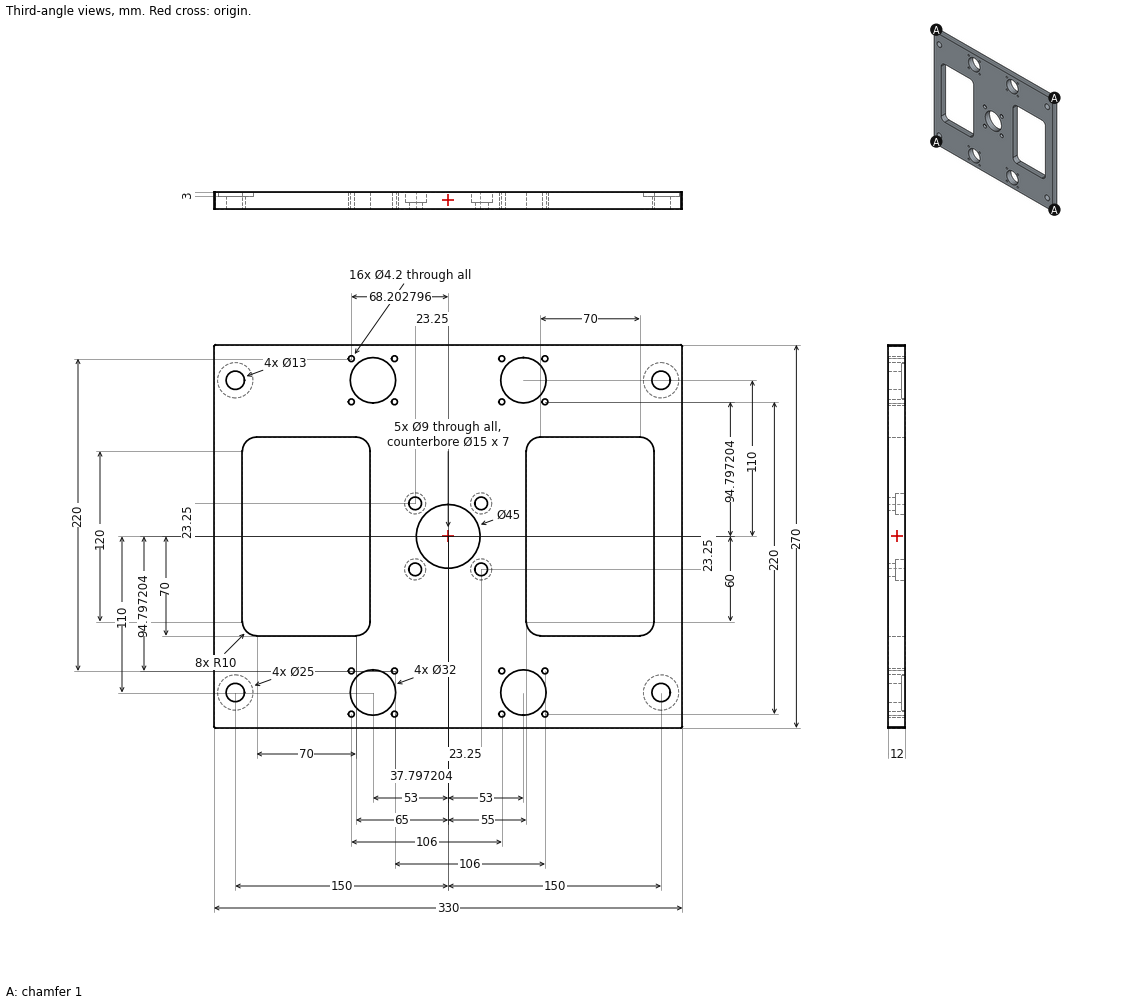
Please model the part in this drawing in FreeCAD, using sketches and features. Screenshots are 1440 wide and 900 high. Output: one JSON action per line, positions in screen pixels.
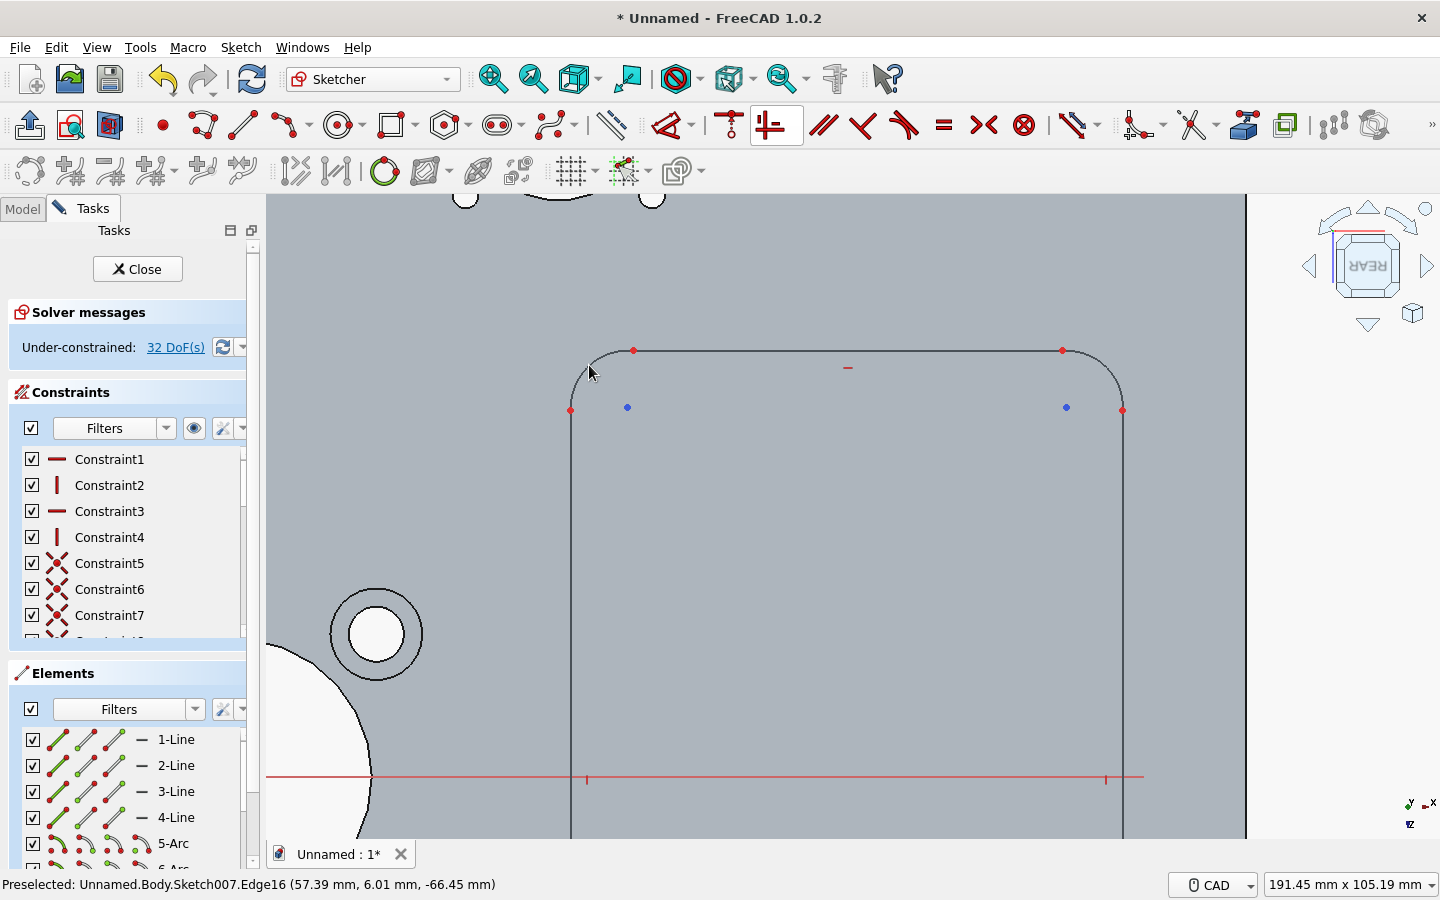
{"action": "scroll", "coordinate": [1105, 365], "scroll_direction": "down", "scroll_amount": 5}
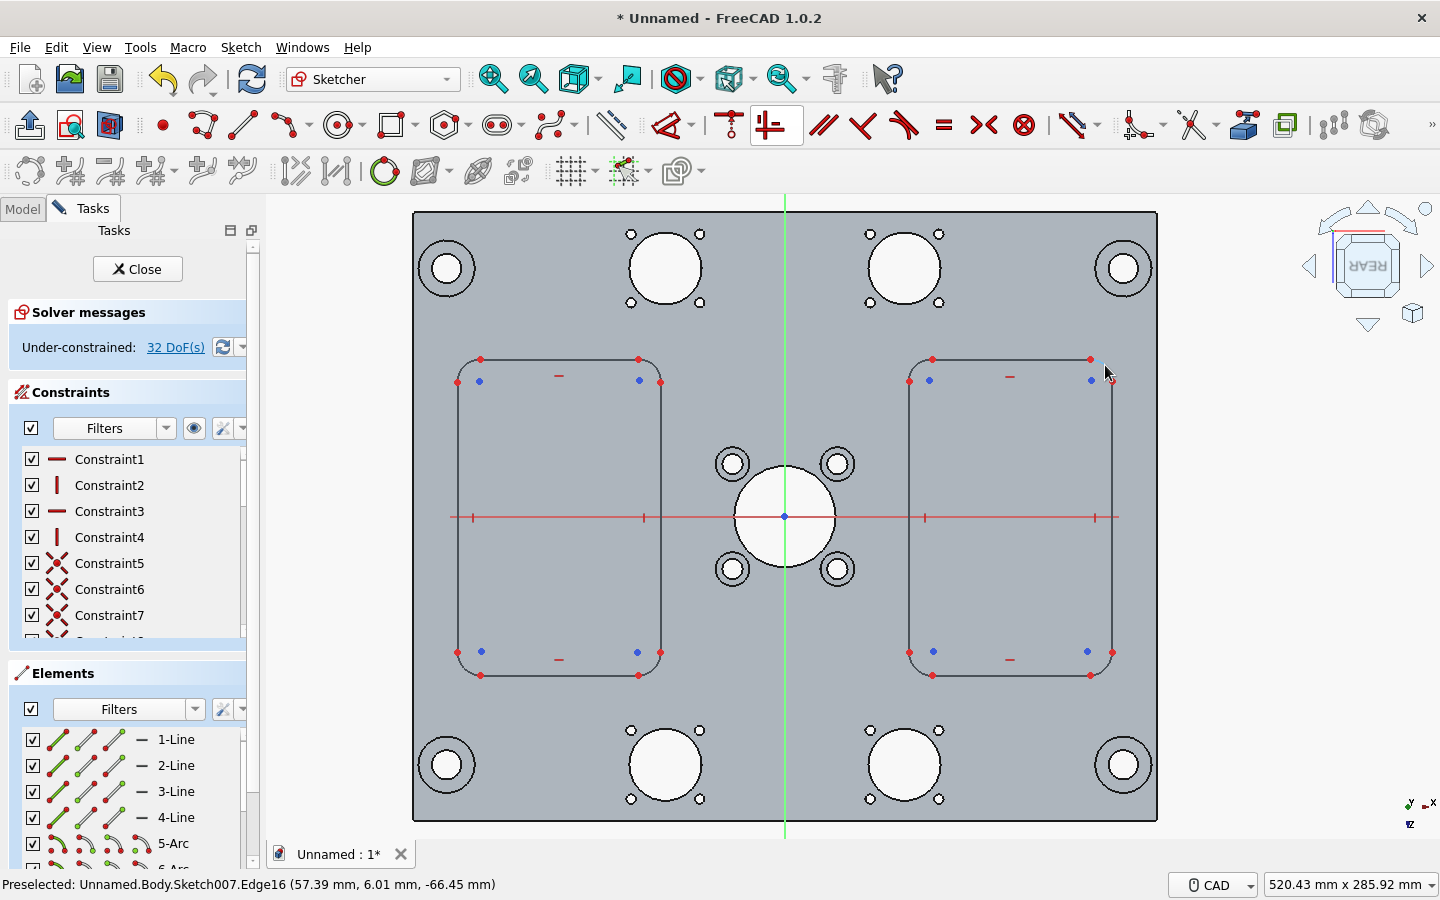
{"action": "left_click", "coordinate": [591, 360]}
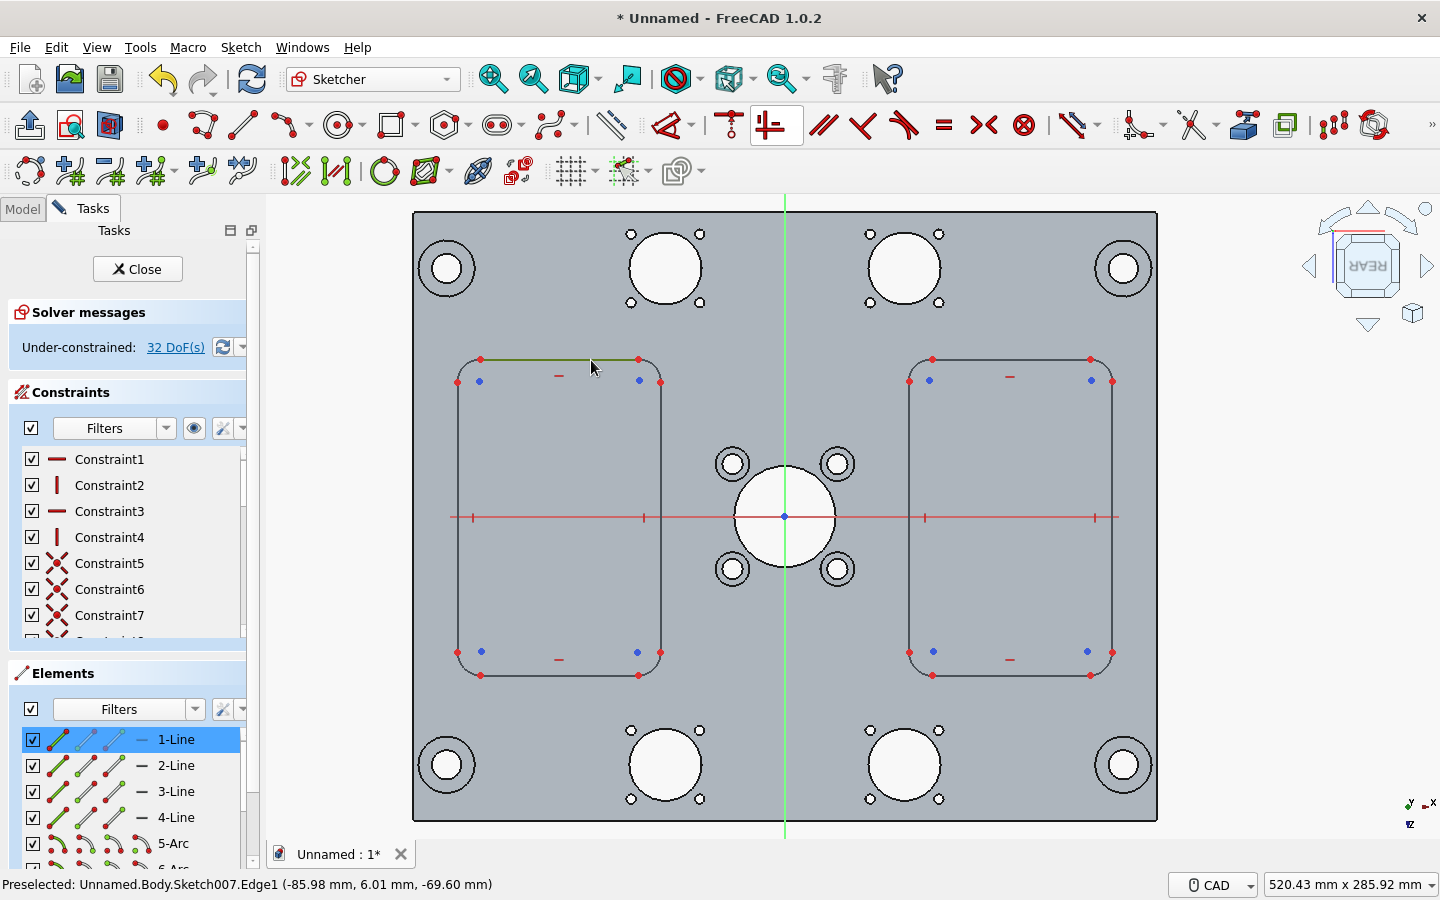
{"action": "scroll", "coordinate": [470, 362], "scroll_direction": "up", "scroll_amount": 2}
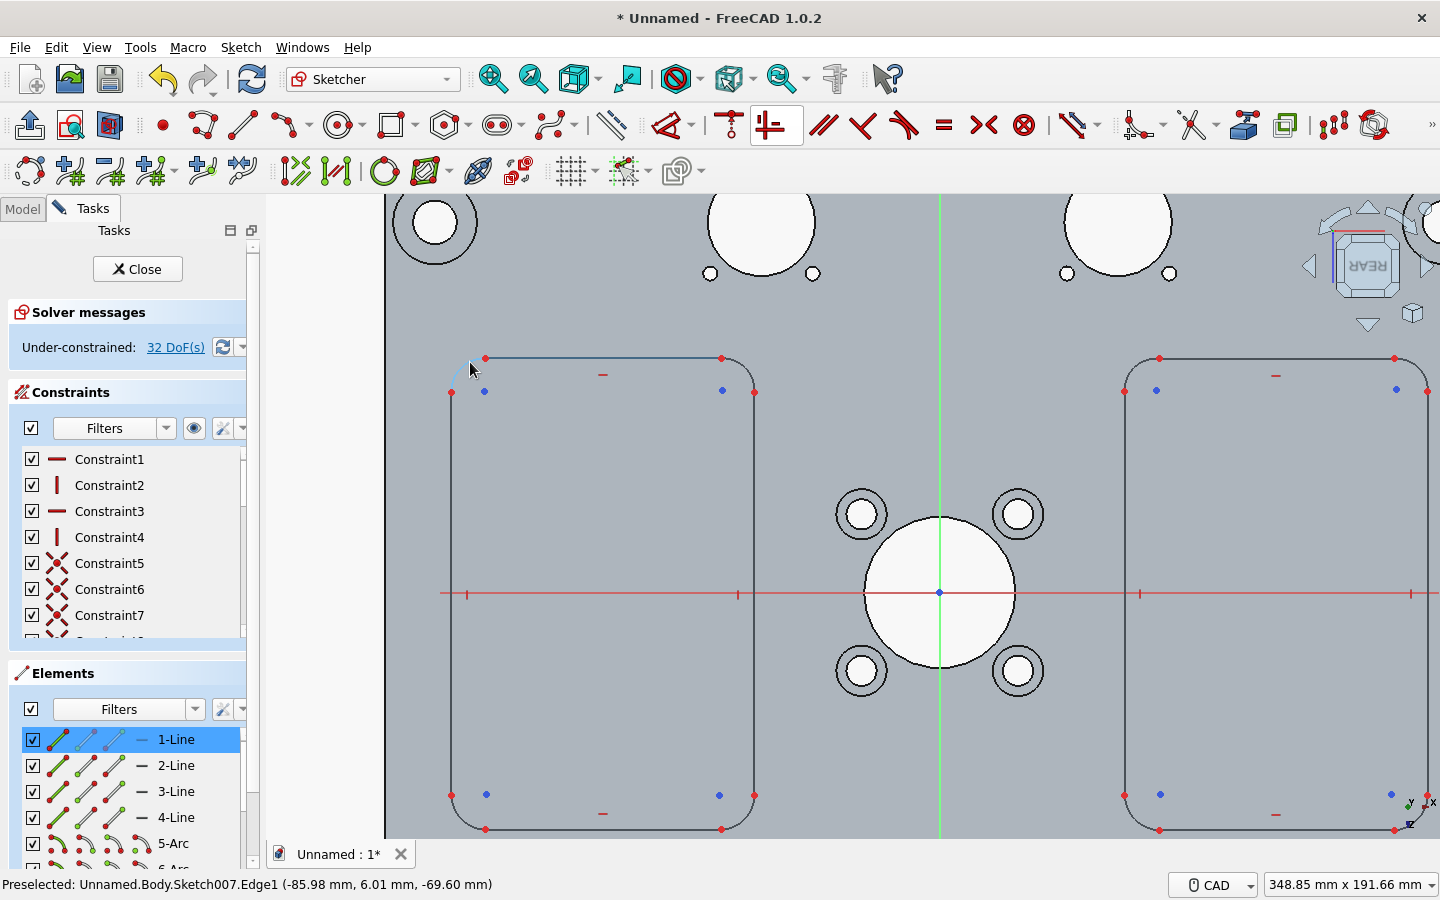
{"action": "left_click", "coordinate": [470, 362]}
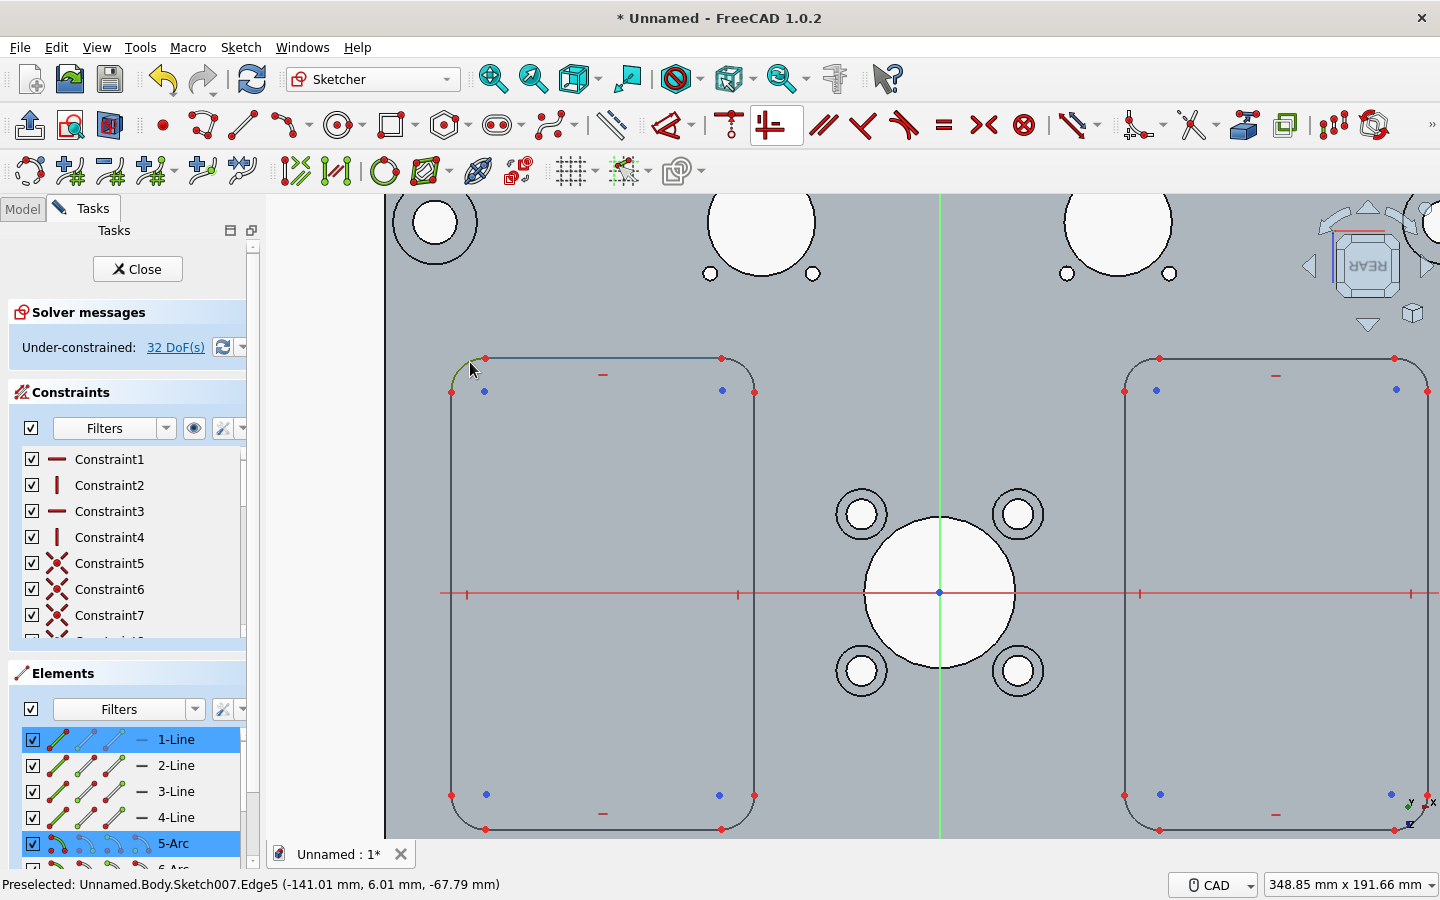
{"action": "left_click", "coordinate": [904, 126]}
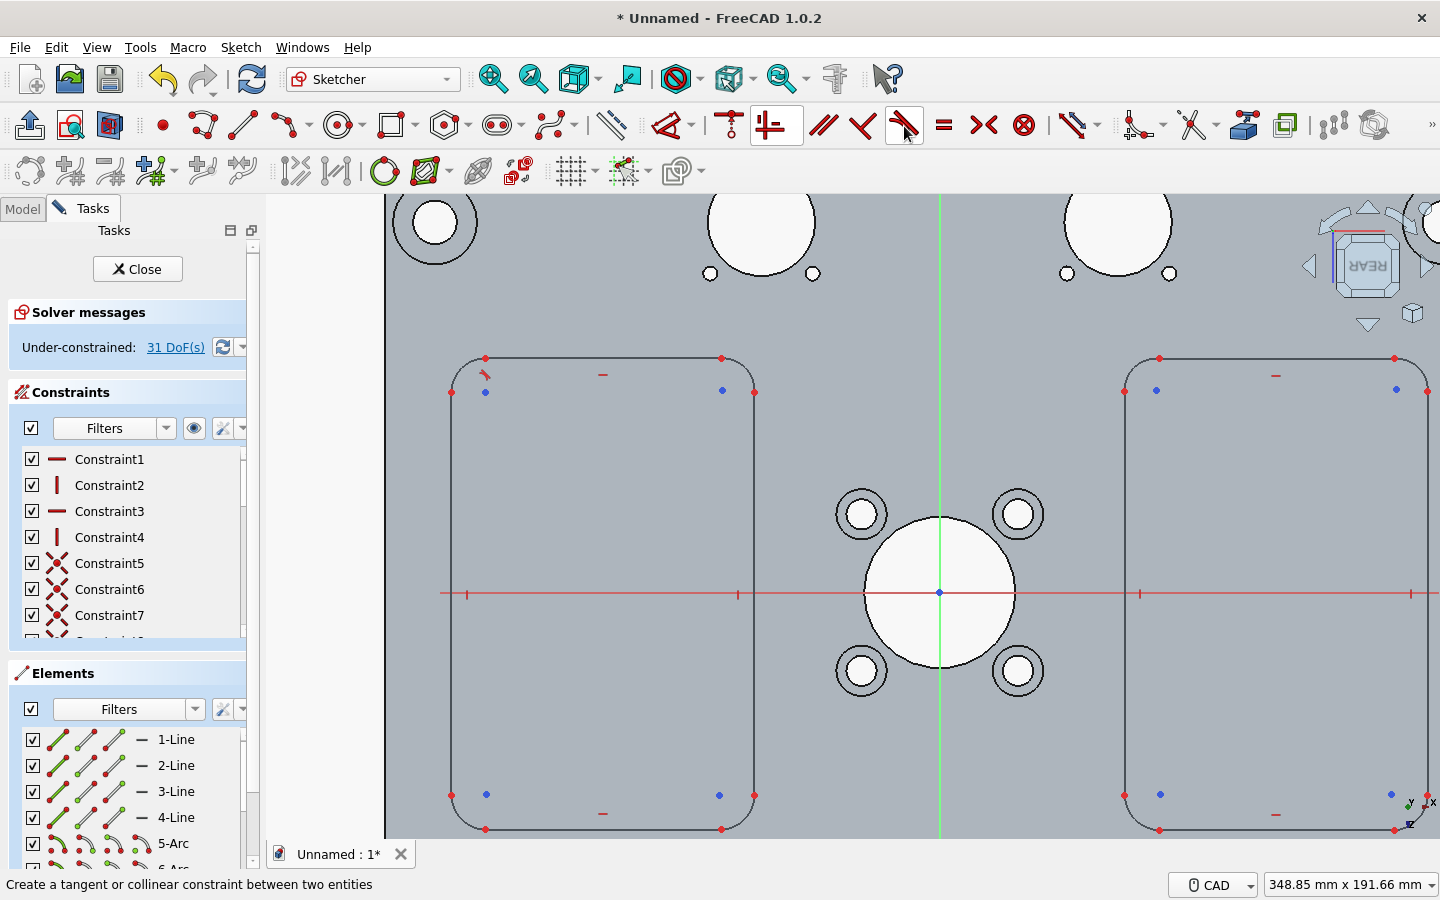
{"action": "left_click", "coordinate": [651, 358]}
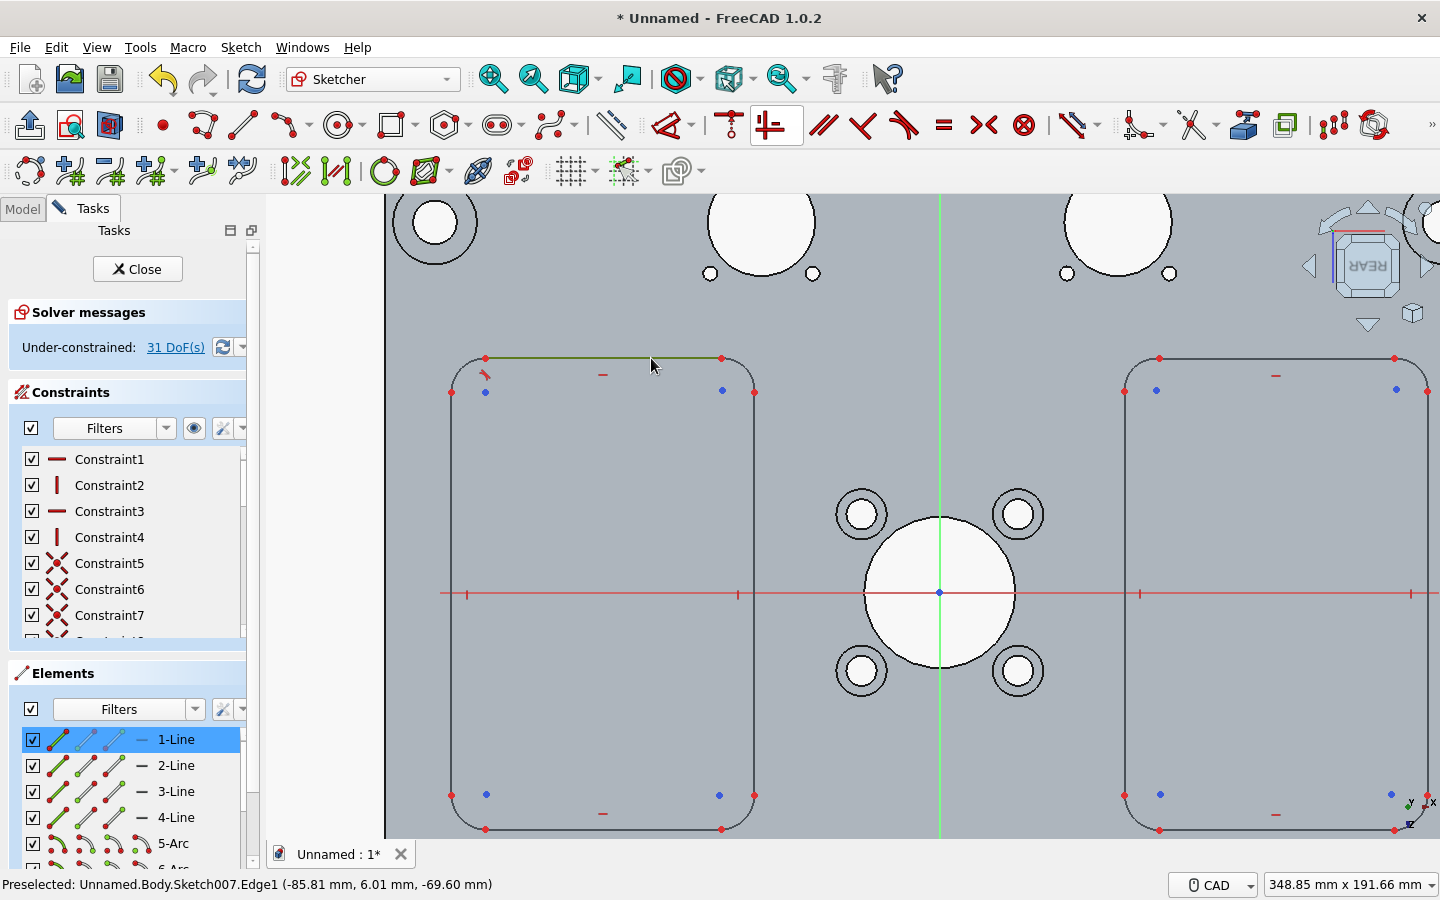
{"action": "left_click", "coordinate": [752, 377]}